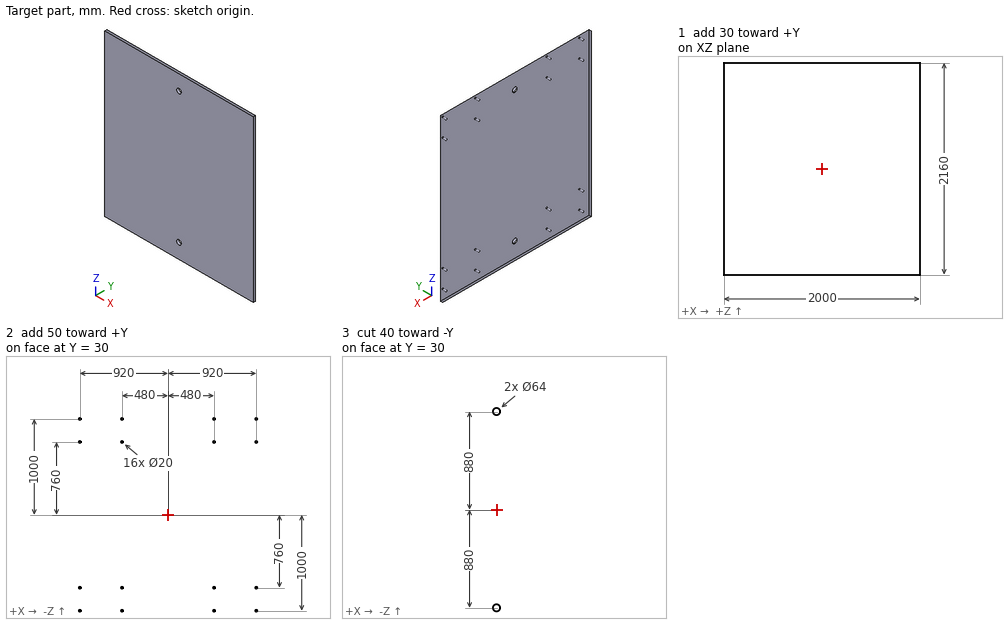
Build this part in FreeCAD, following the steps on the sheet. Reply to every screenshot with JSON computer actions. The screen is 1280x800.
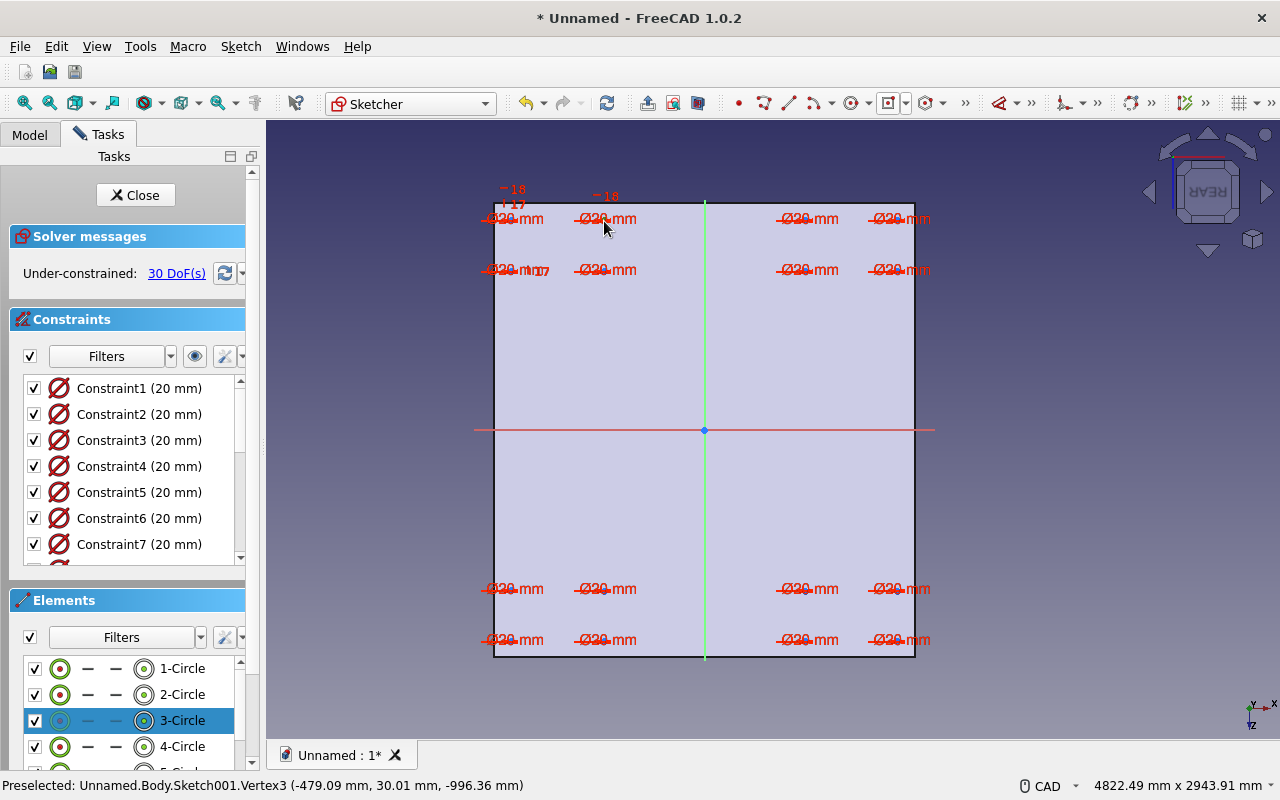
{"action": "left_click", "coordinate": [604, 272]}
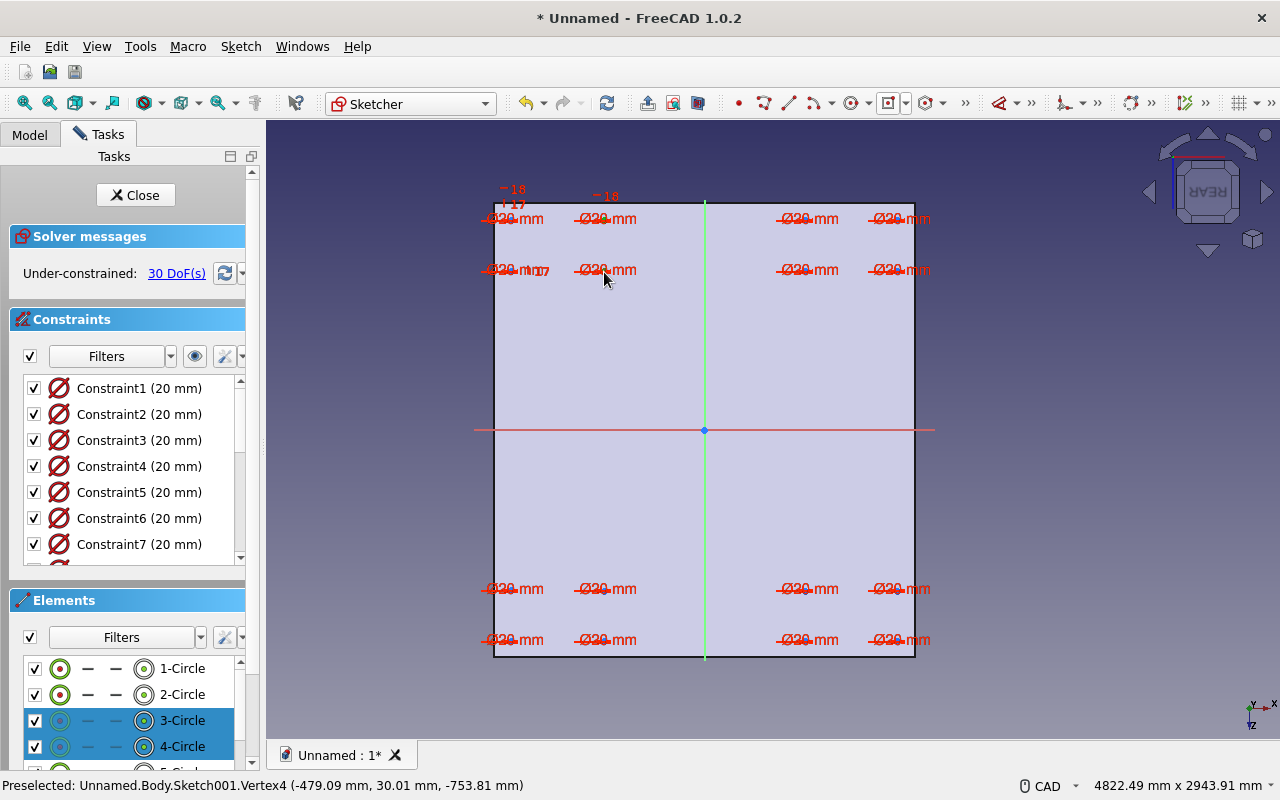
{"action": "key", "text": "v"}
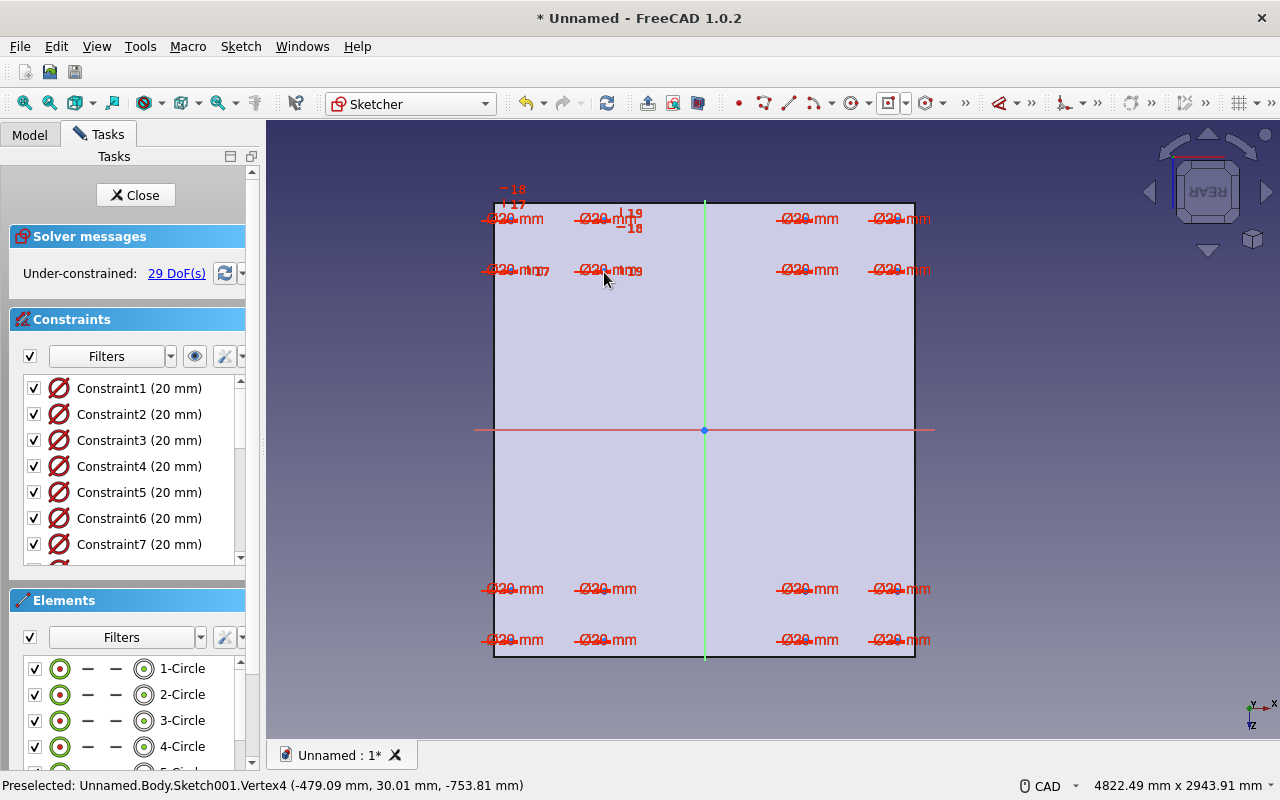
{"action": "left_click", "coordinate": [511, 272]}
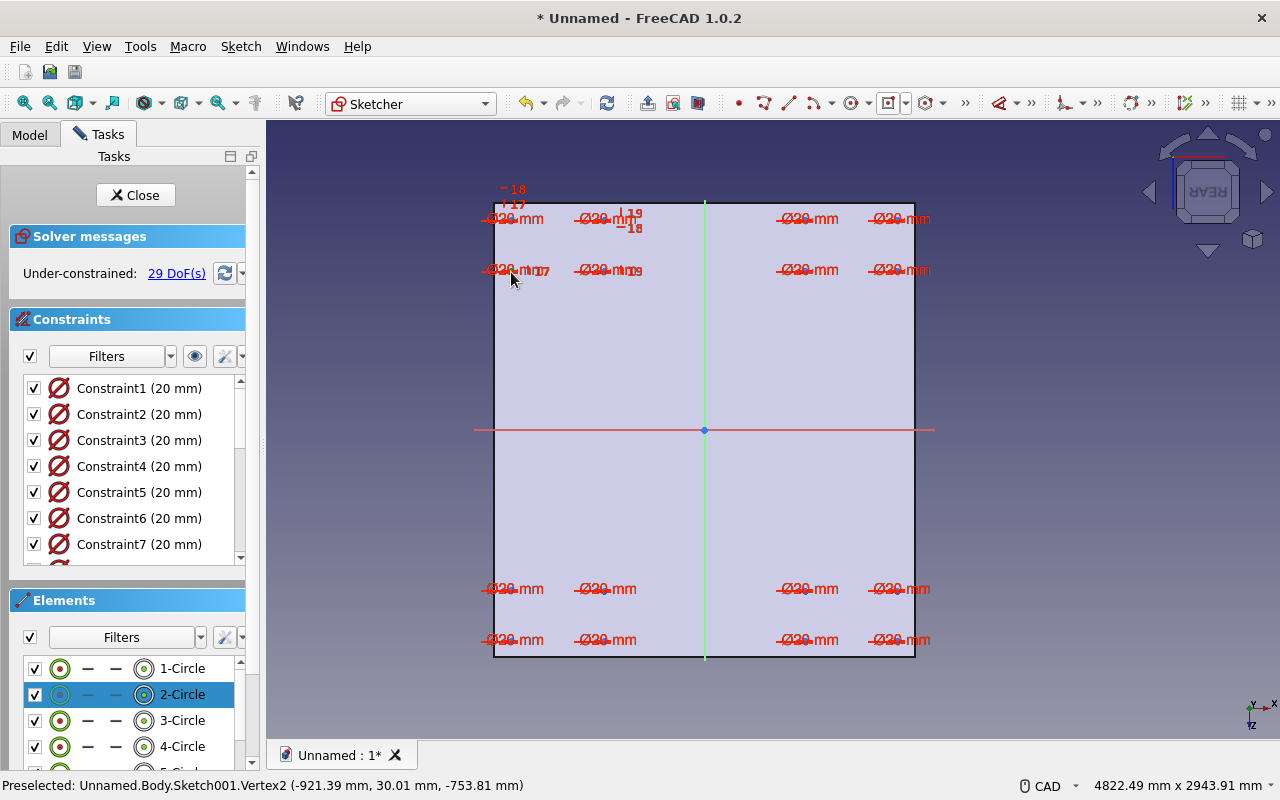
{"action": "left_click", "coordinate": [604, 272]}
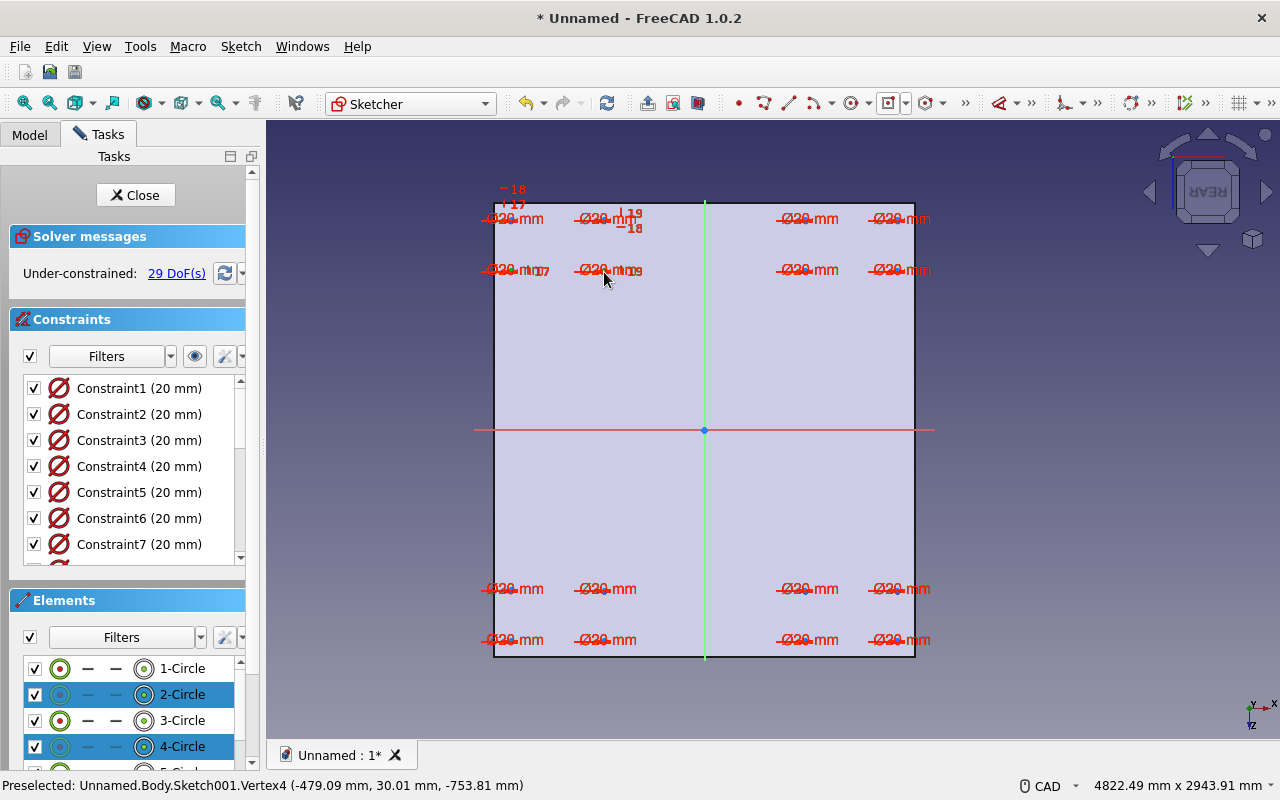
{"action": "key", "text": "h"}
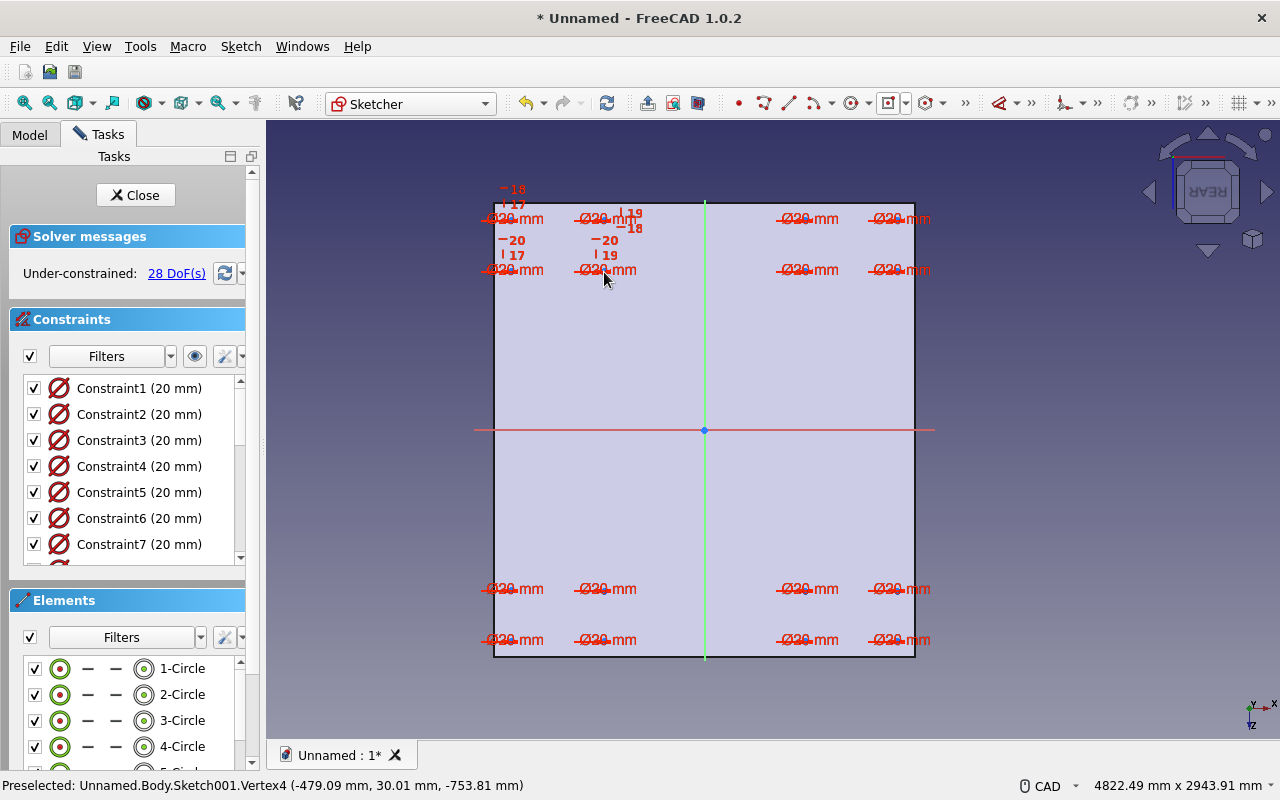
{"action": "left_click", "coordinate": [604, 272]}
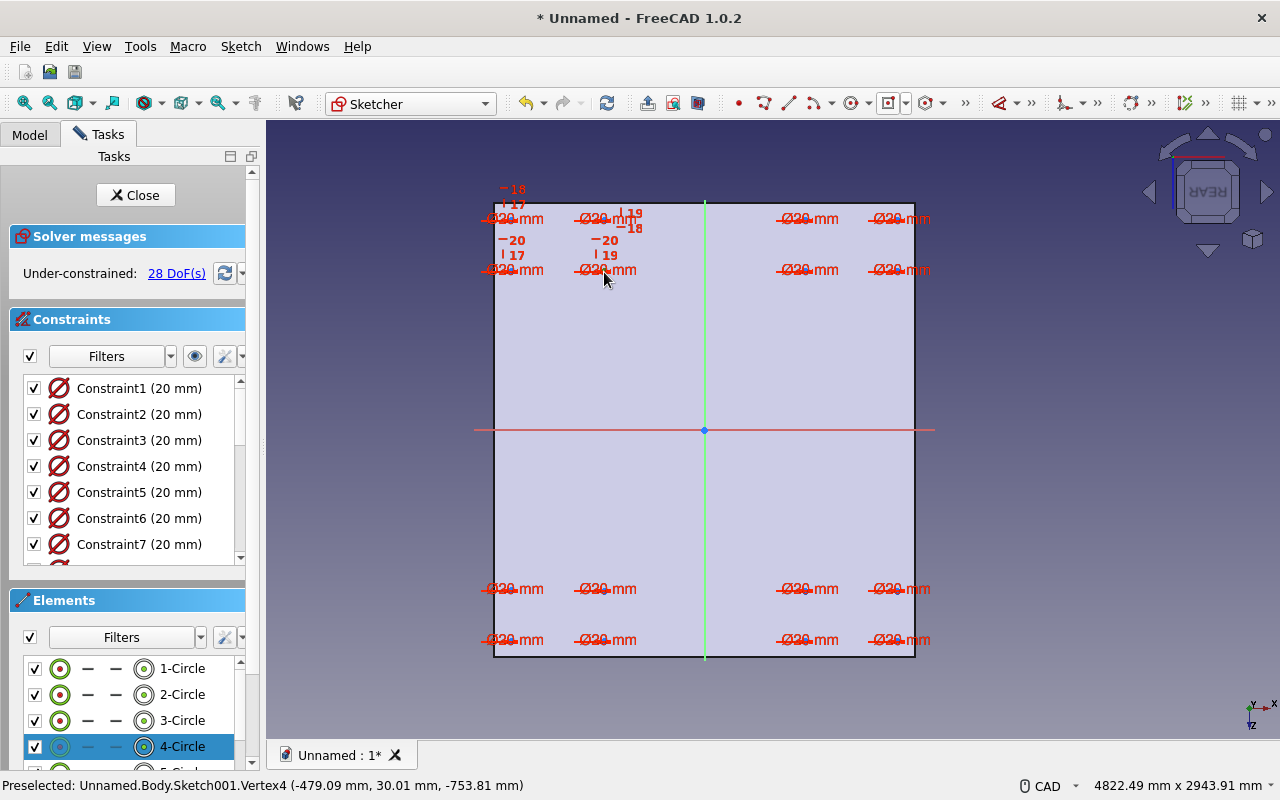
{"action": "left_click", "coordinate": [806, 272]}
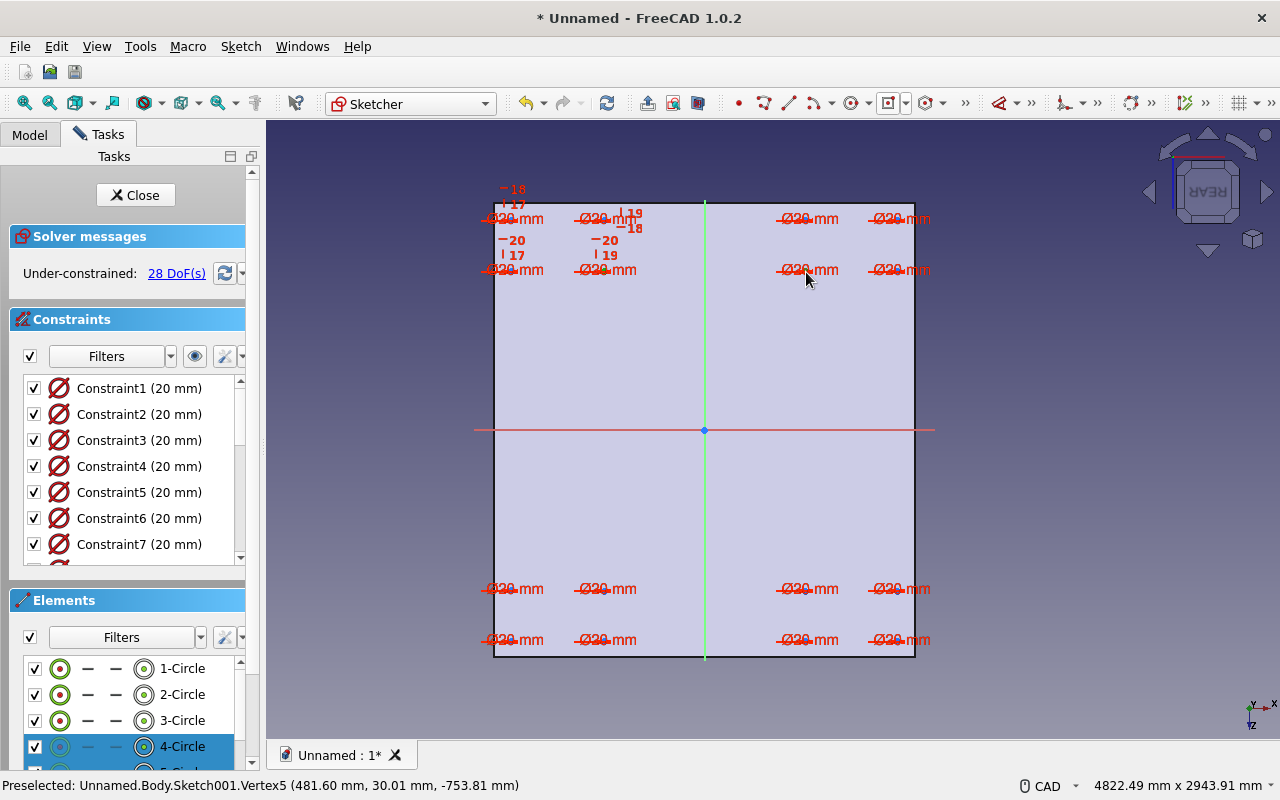
{"action": "key", "text": "h"}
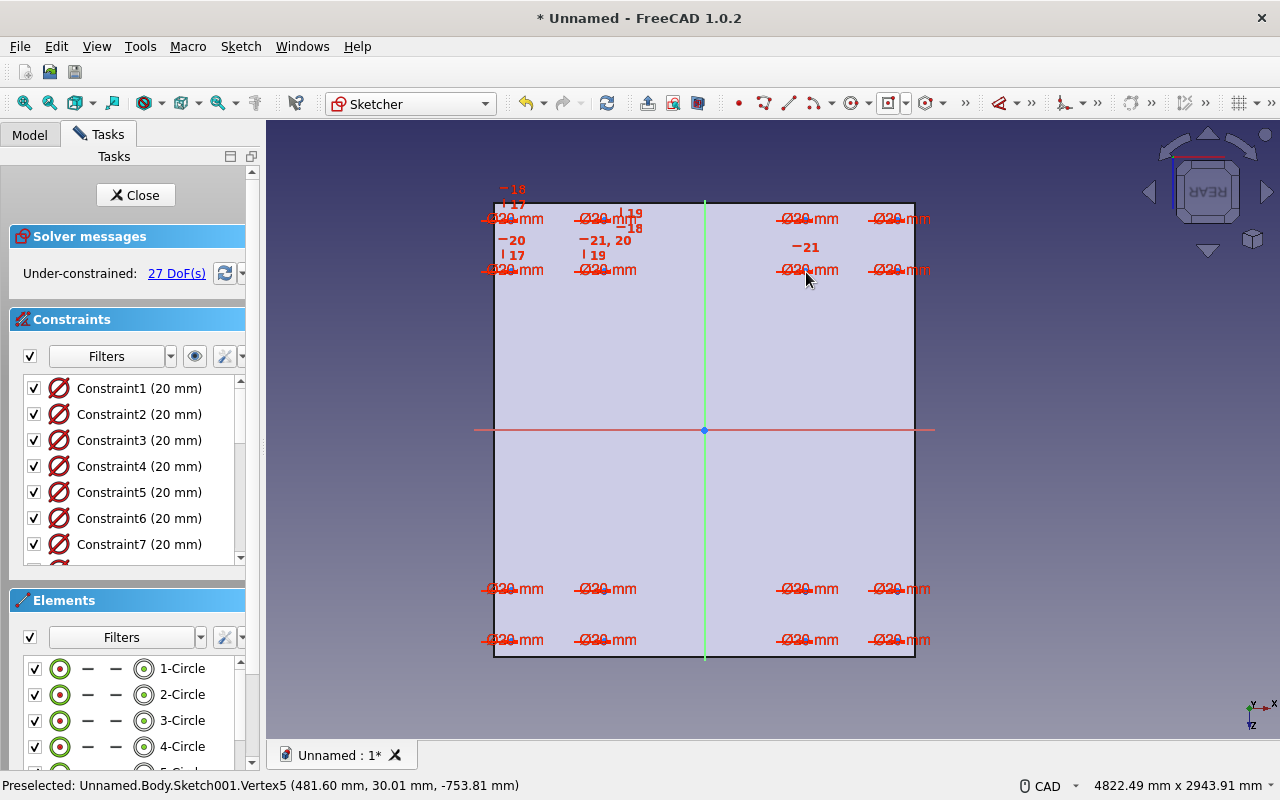
{"action": "left_click", "coordinate": [806, 272]}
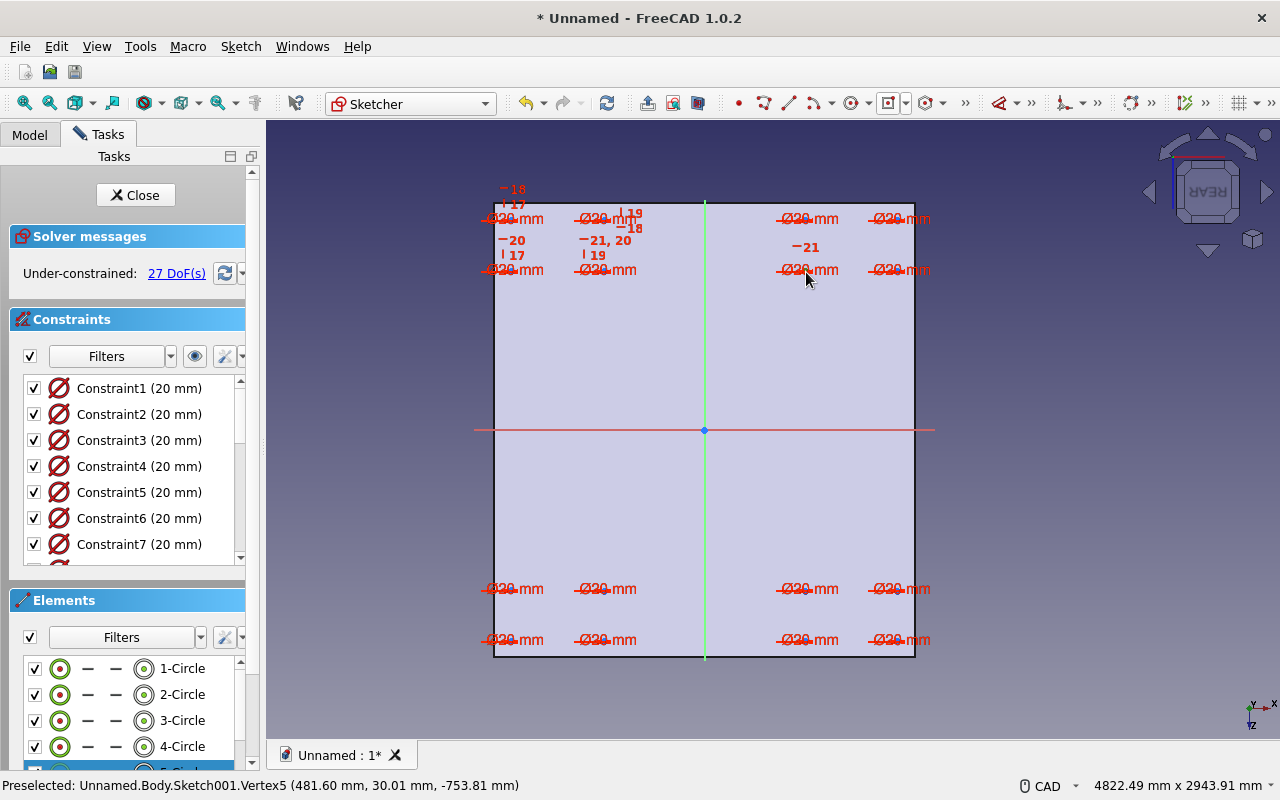
{"action": "left_click", "coordinate": [806, 221]}